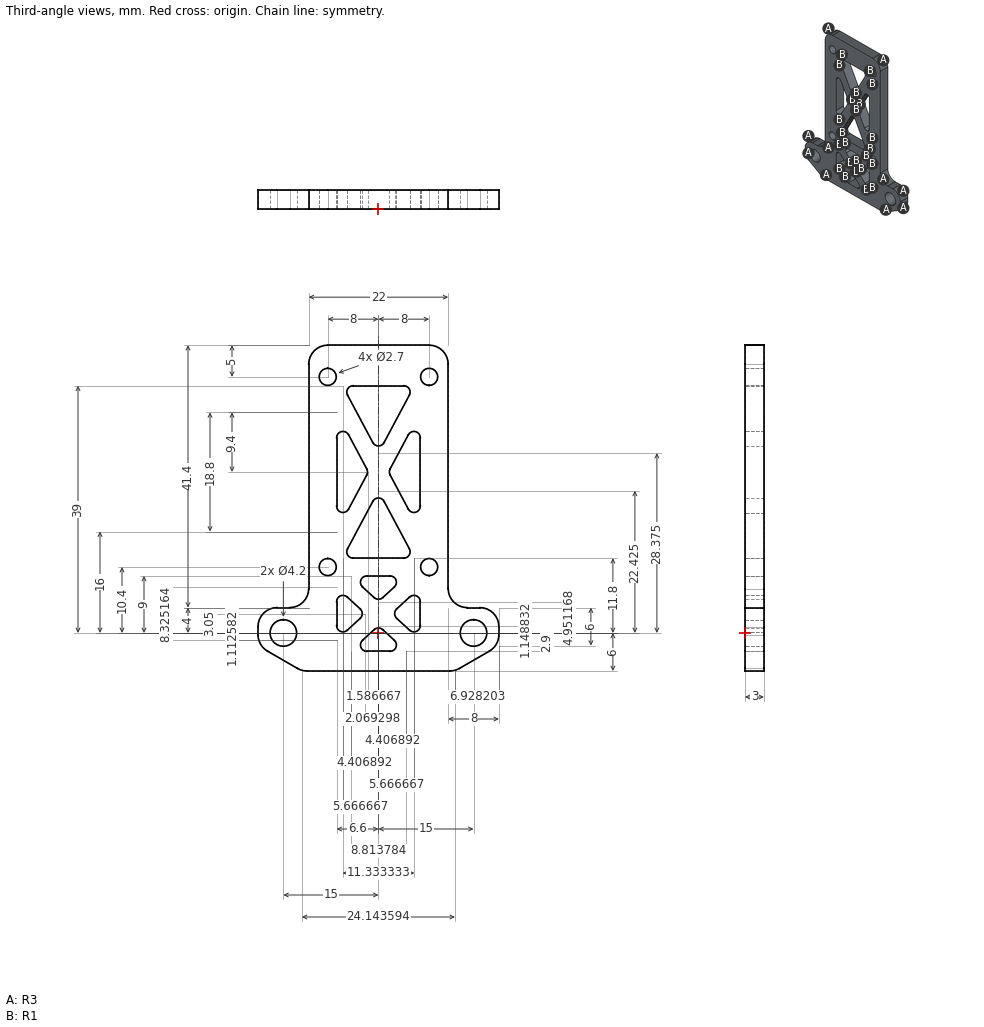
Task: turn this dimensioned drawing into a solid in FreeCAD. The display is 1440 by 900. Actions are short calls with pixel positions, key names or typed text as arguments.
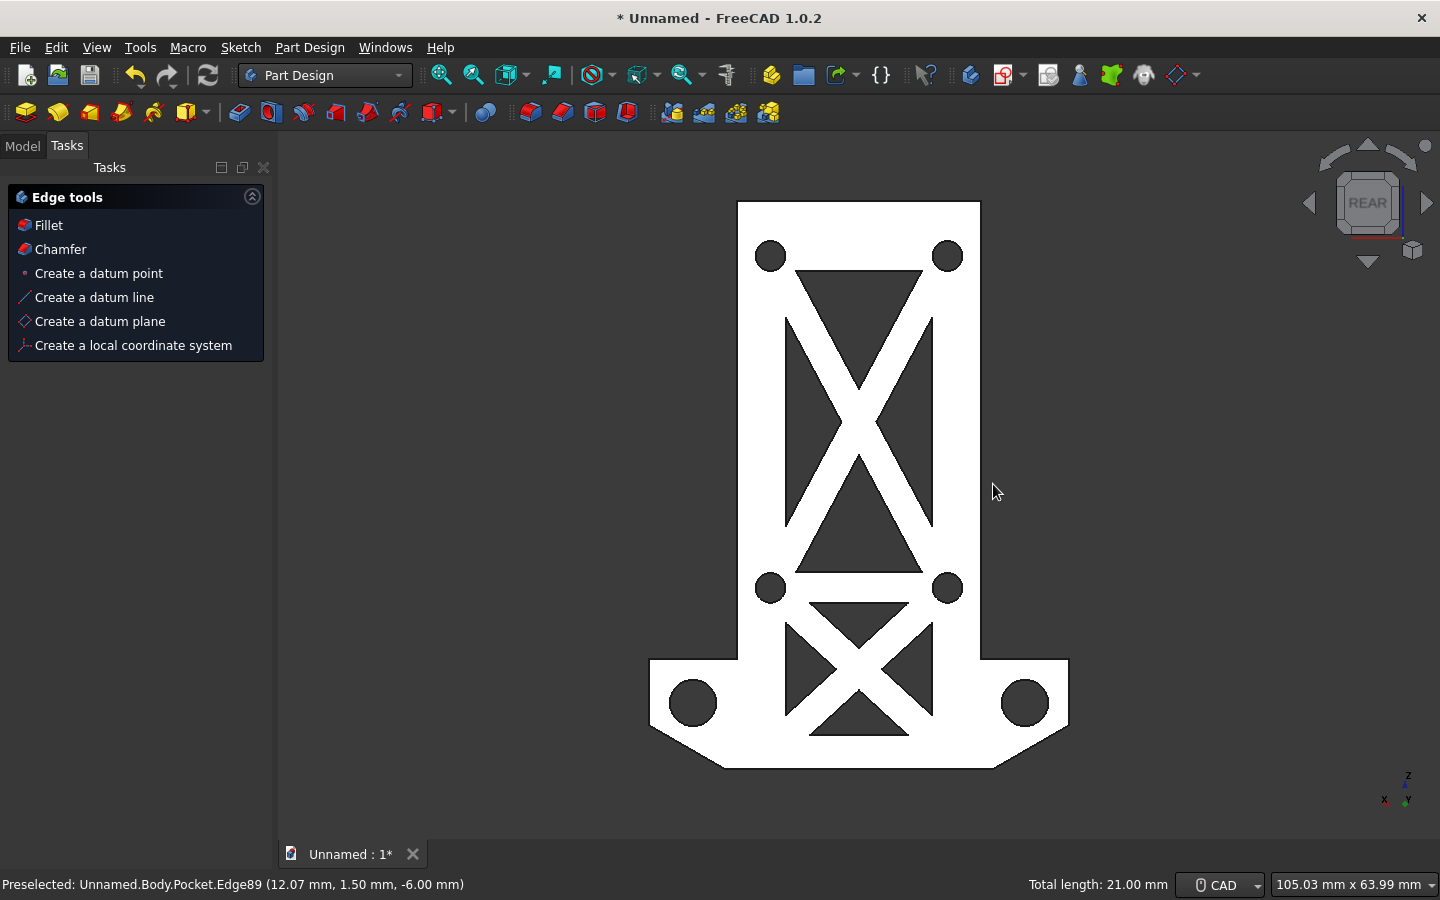
key(6)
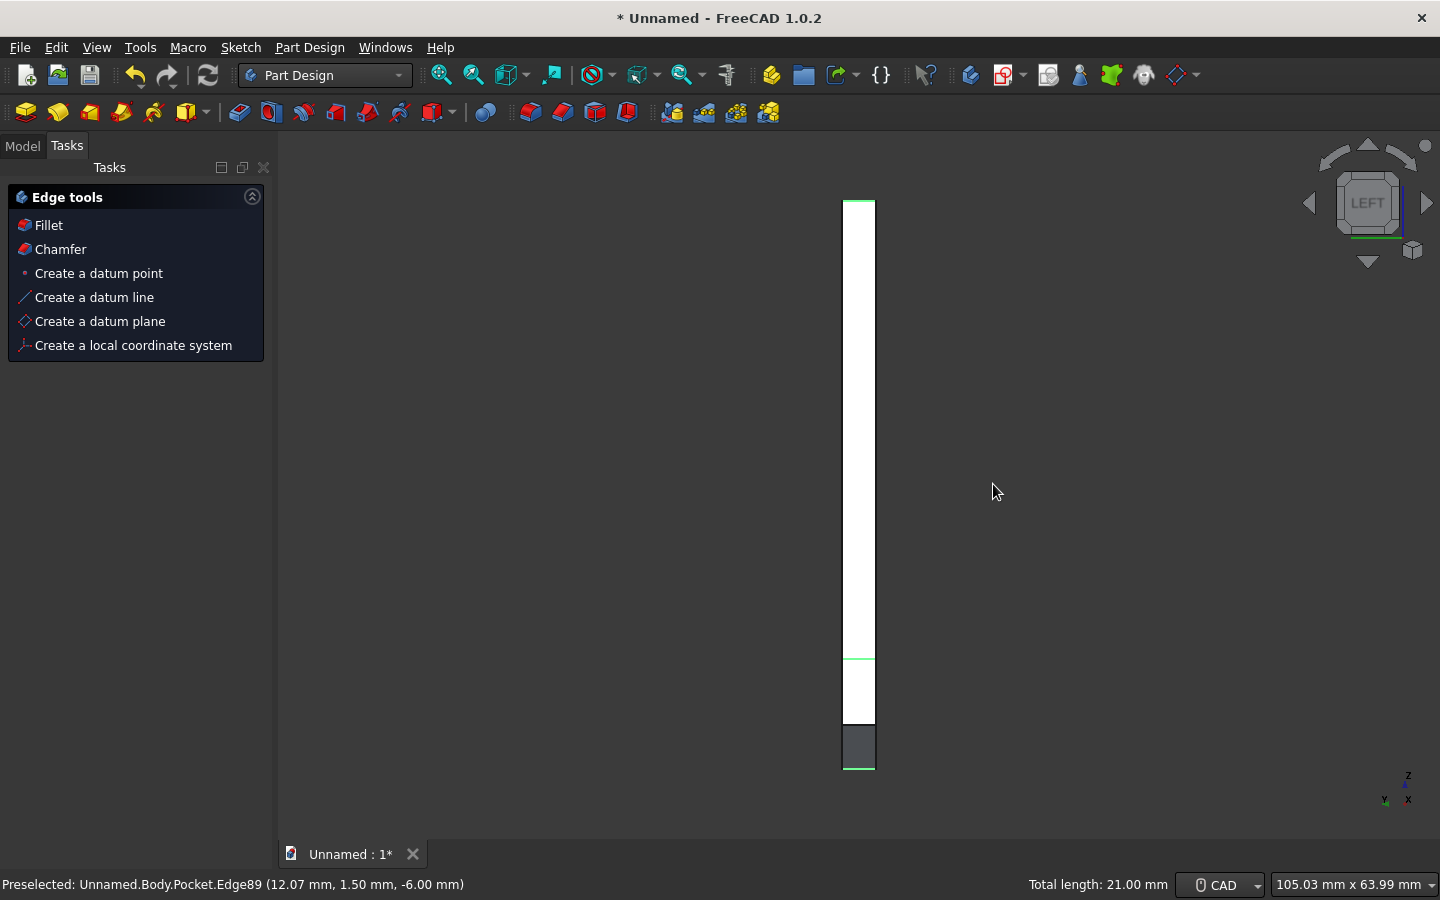
click(859, 724, ctrl)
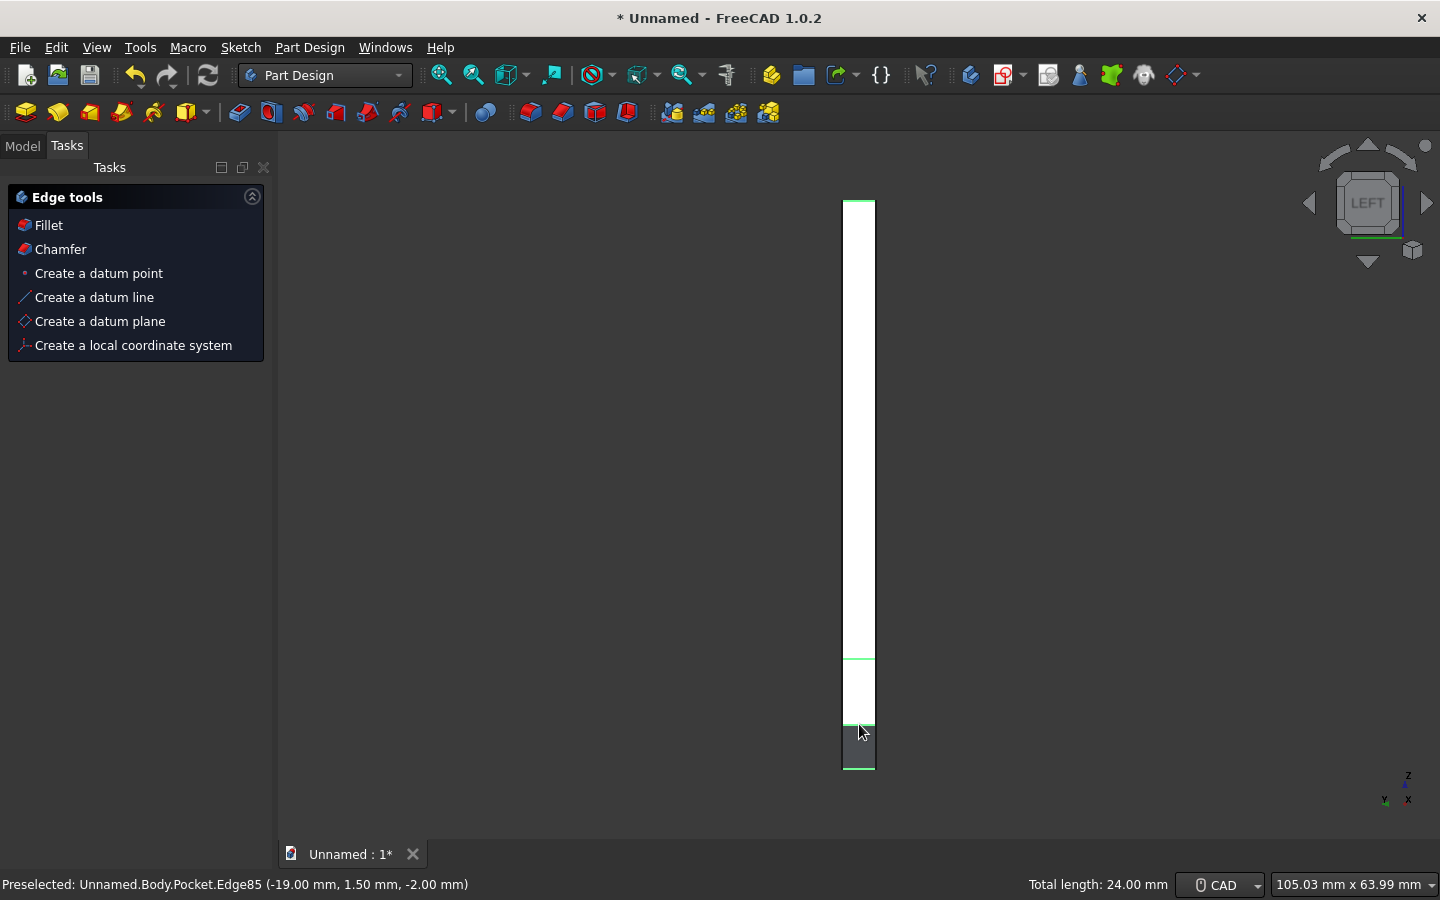
key(v)
key(3)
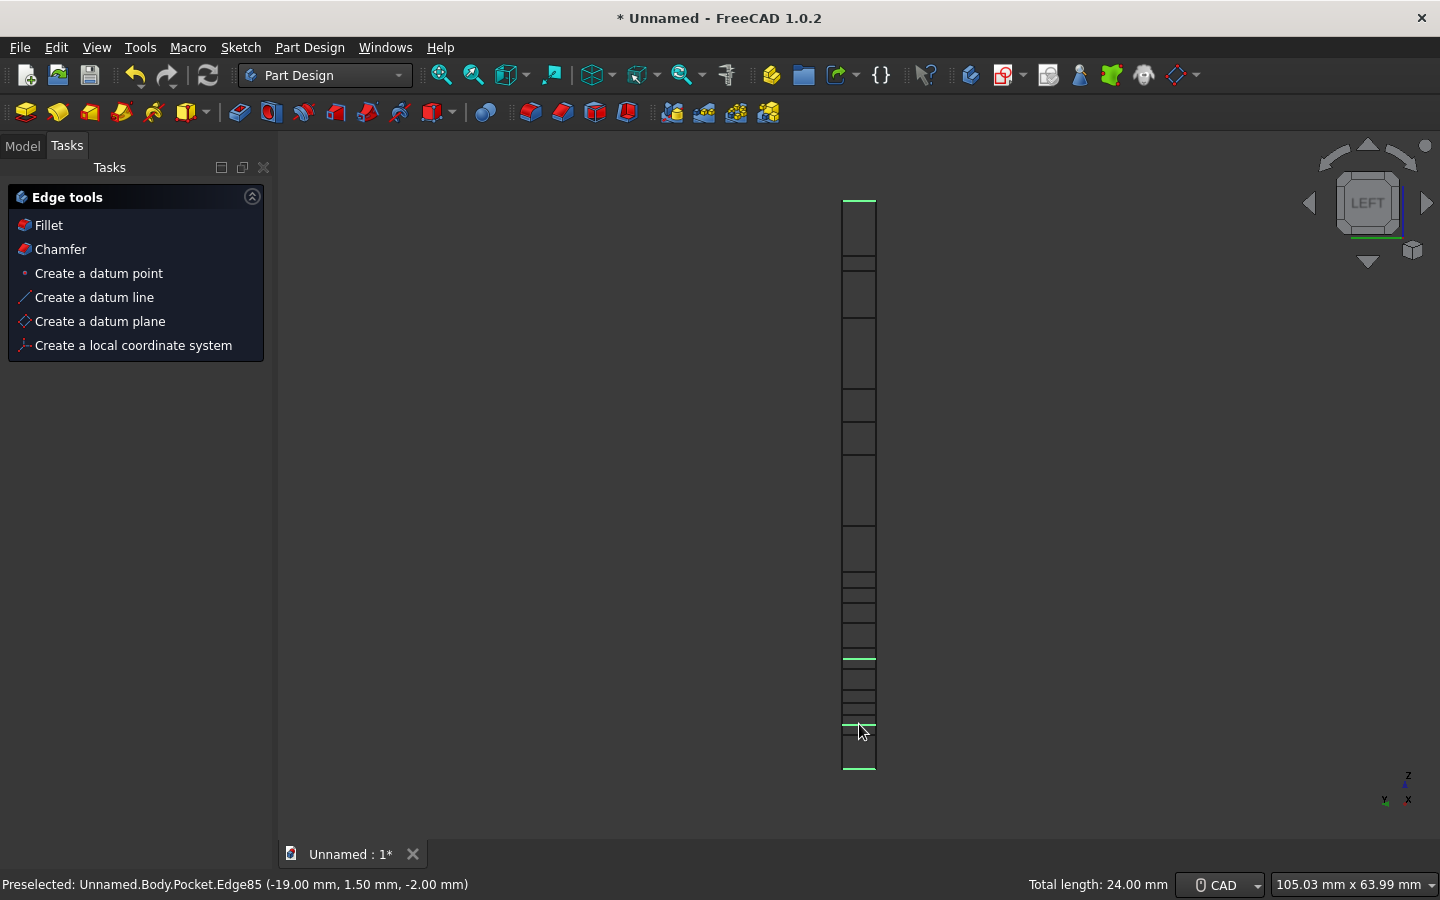
key(0)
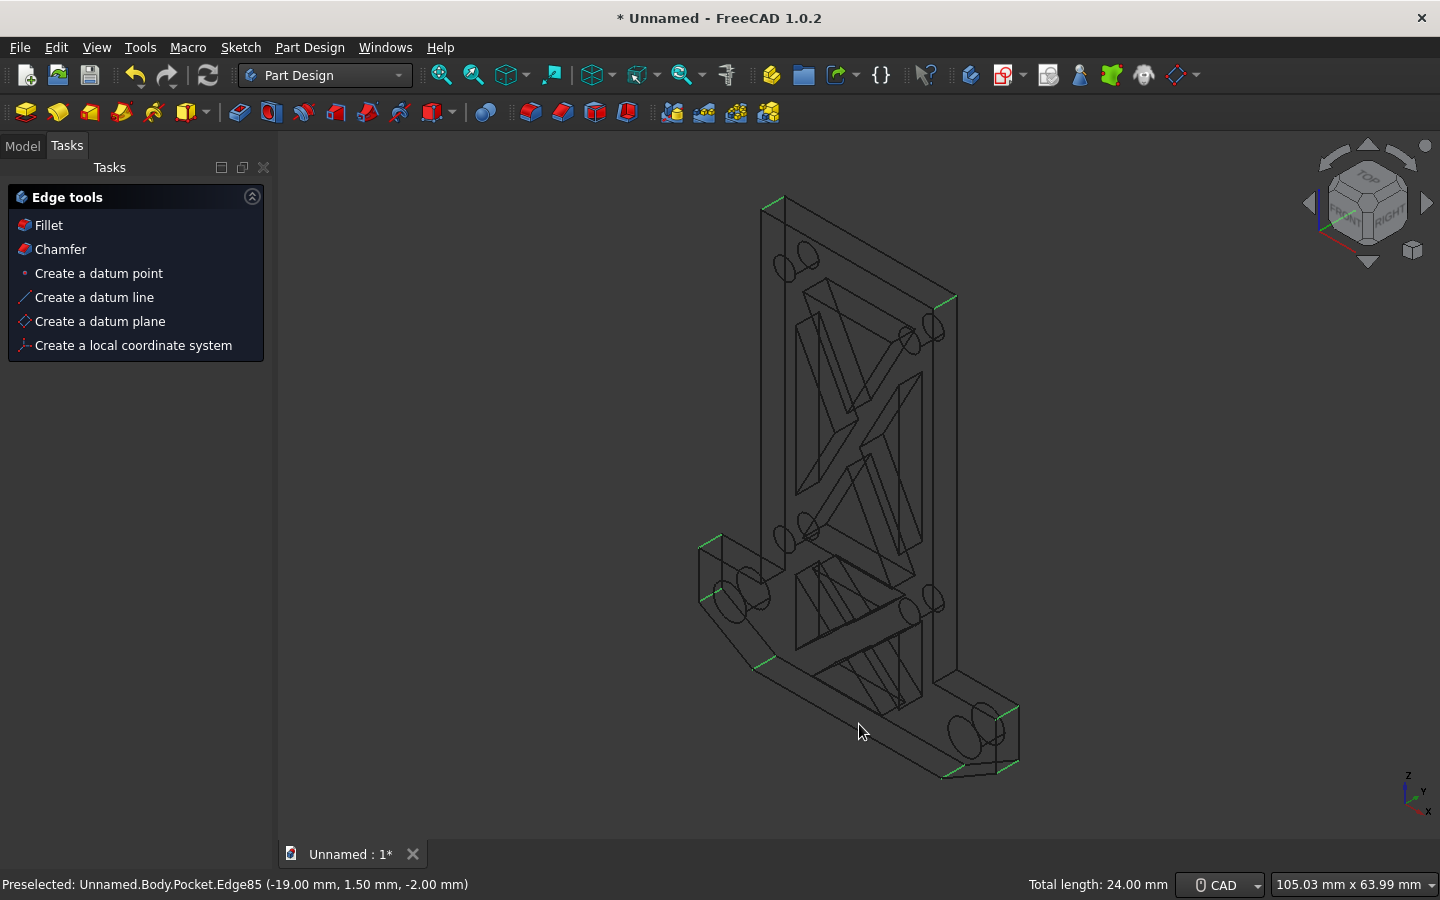
click(945, 676, ctrl)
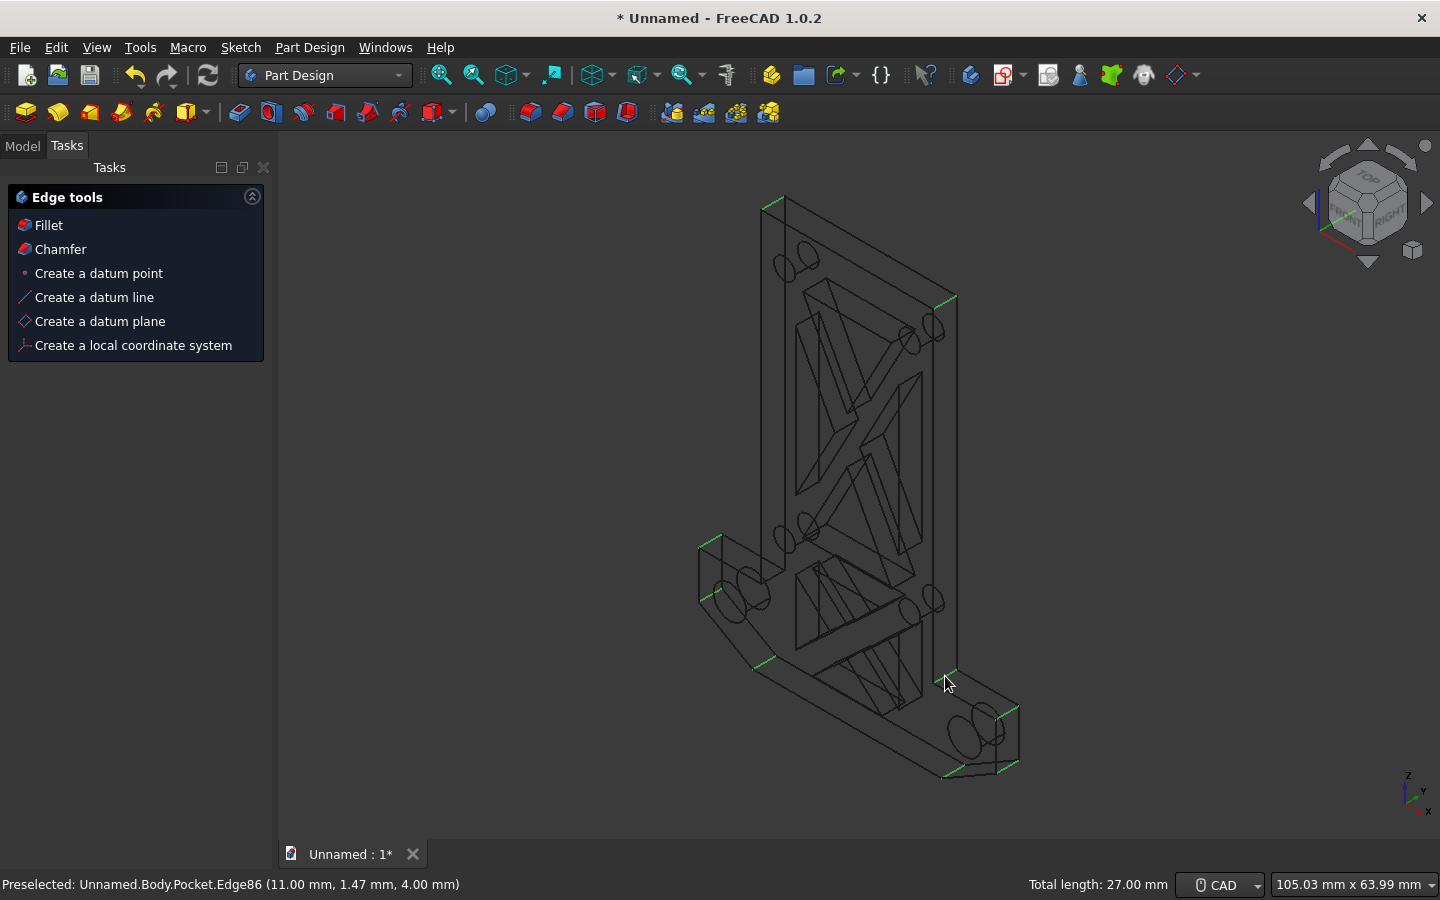
click(773, 576, ctrl)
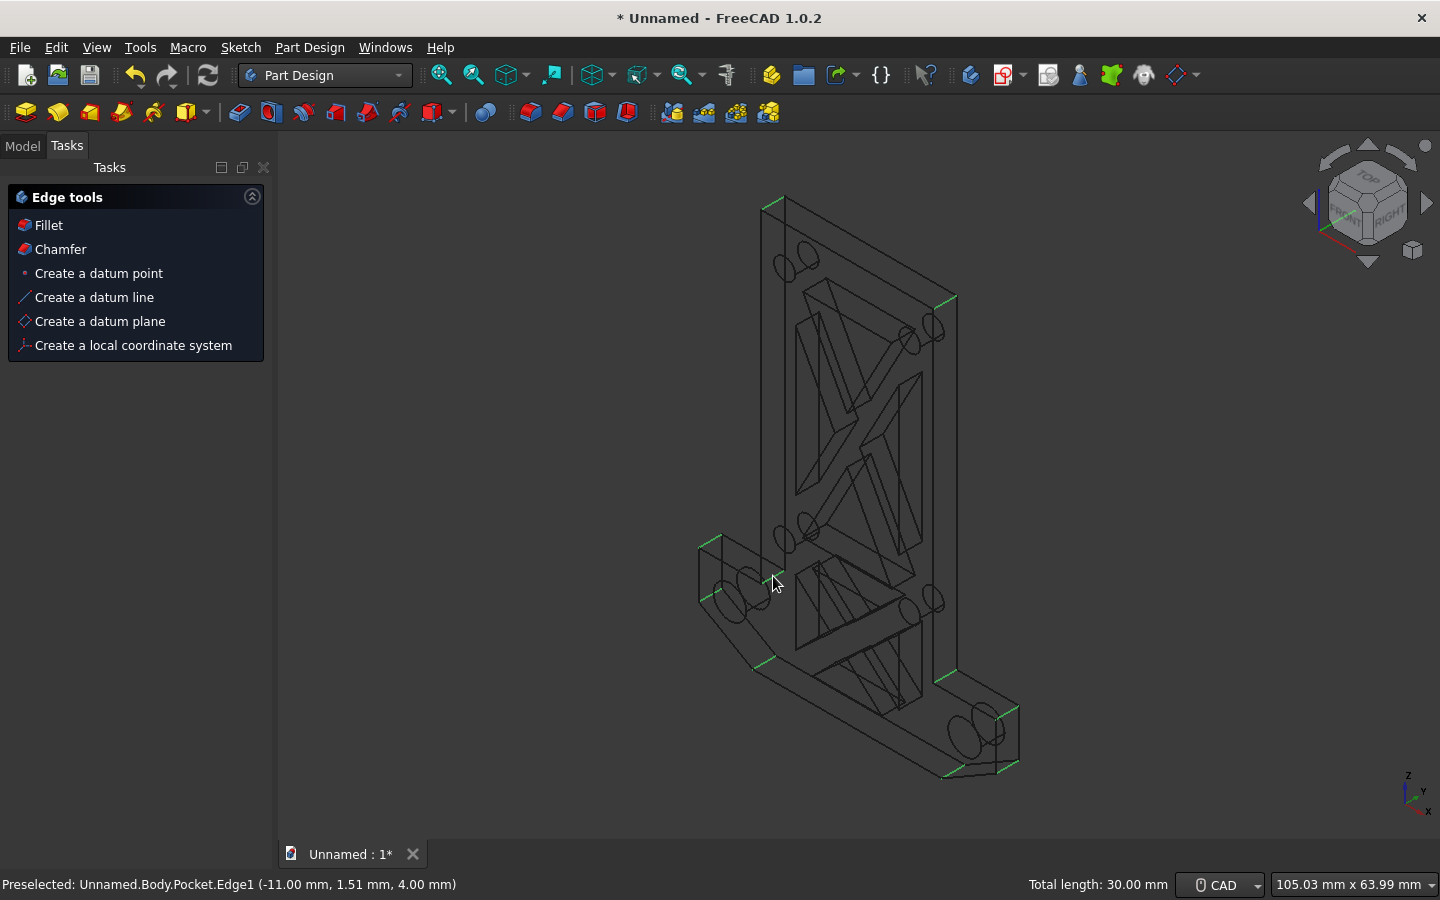
key(v)
key(1)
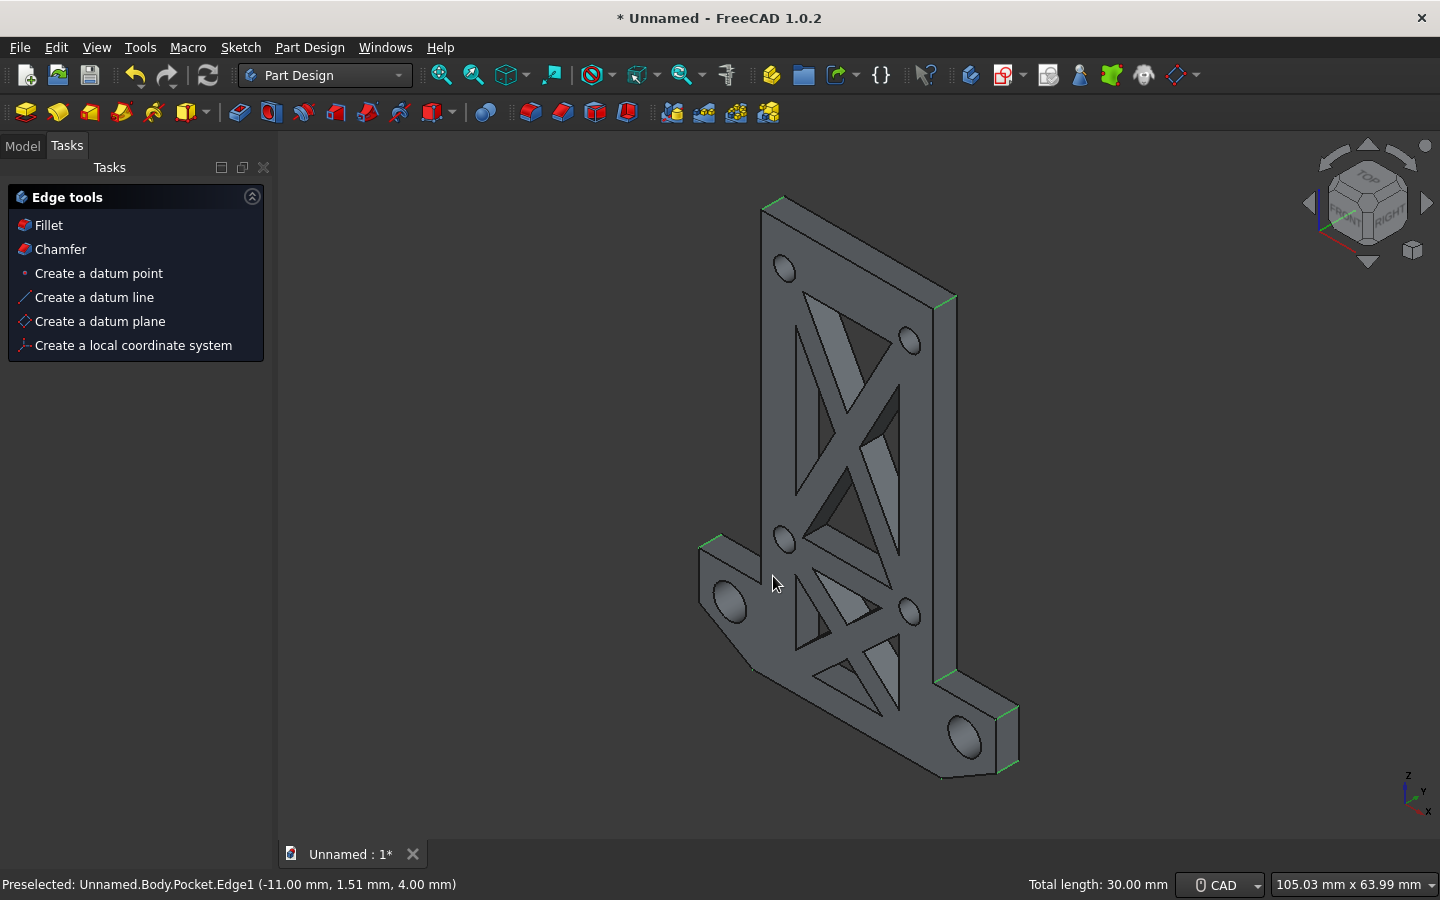
click(532, 112)